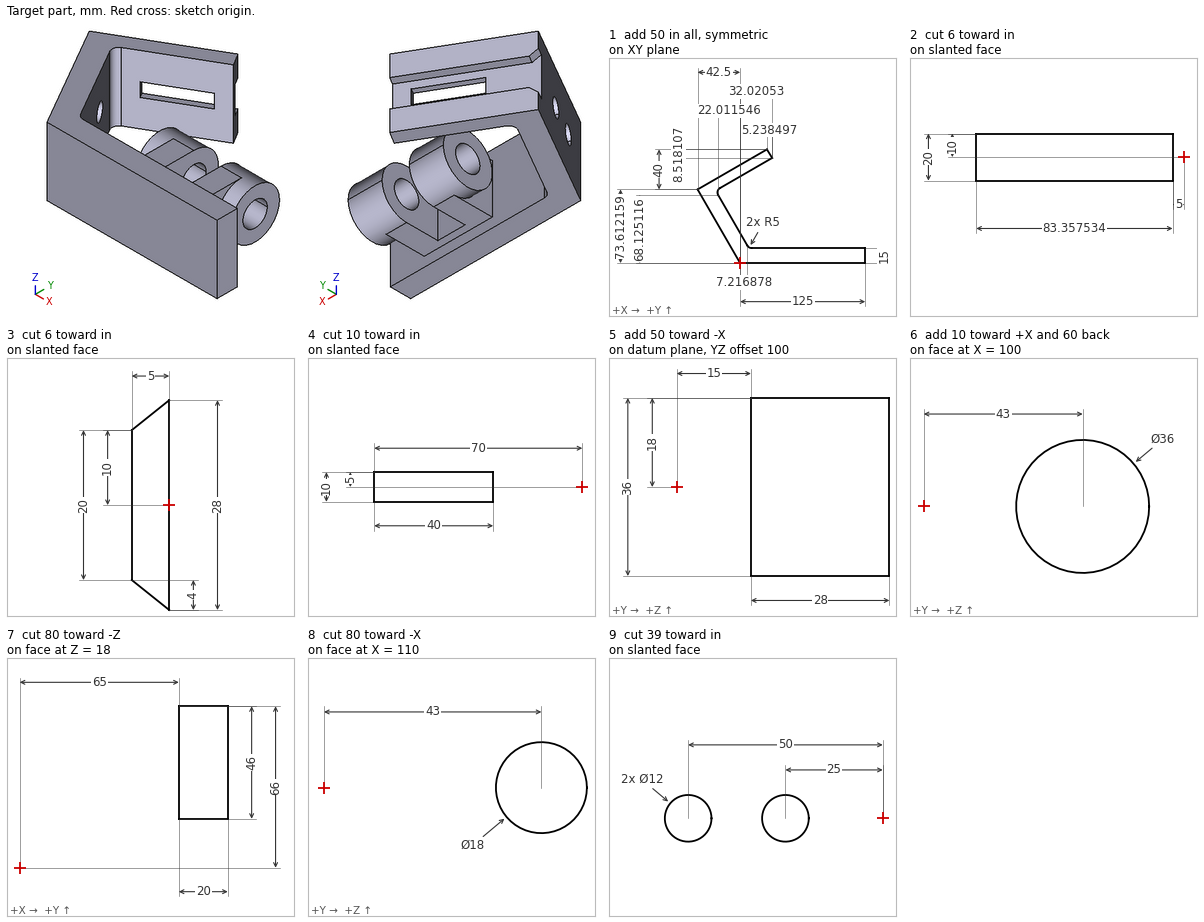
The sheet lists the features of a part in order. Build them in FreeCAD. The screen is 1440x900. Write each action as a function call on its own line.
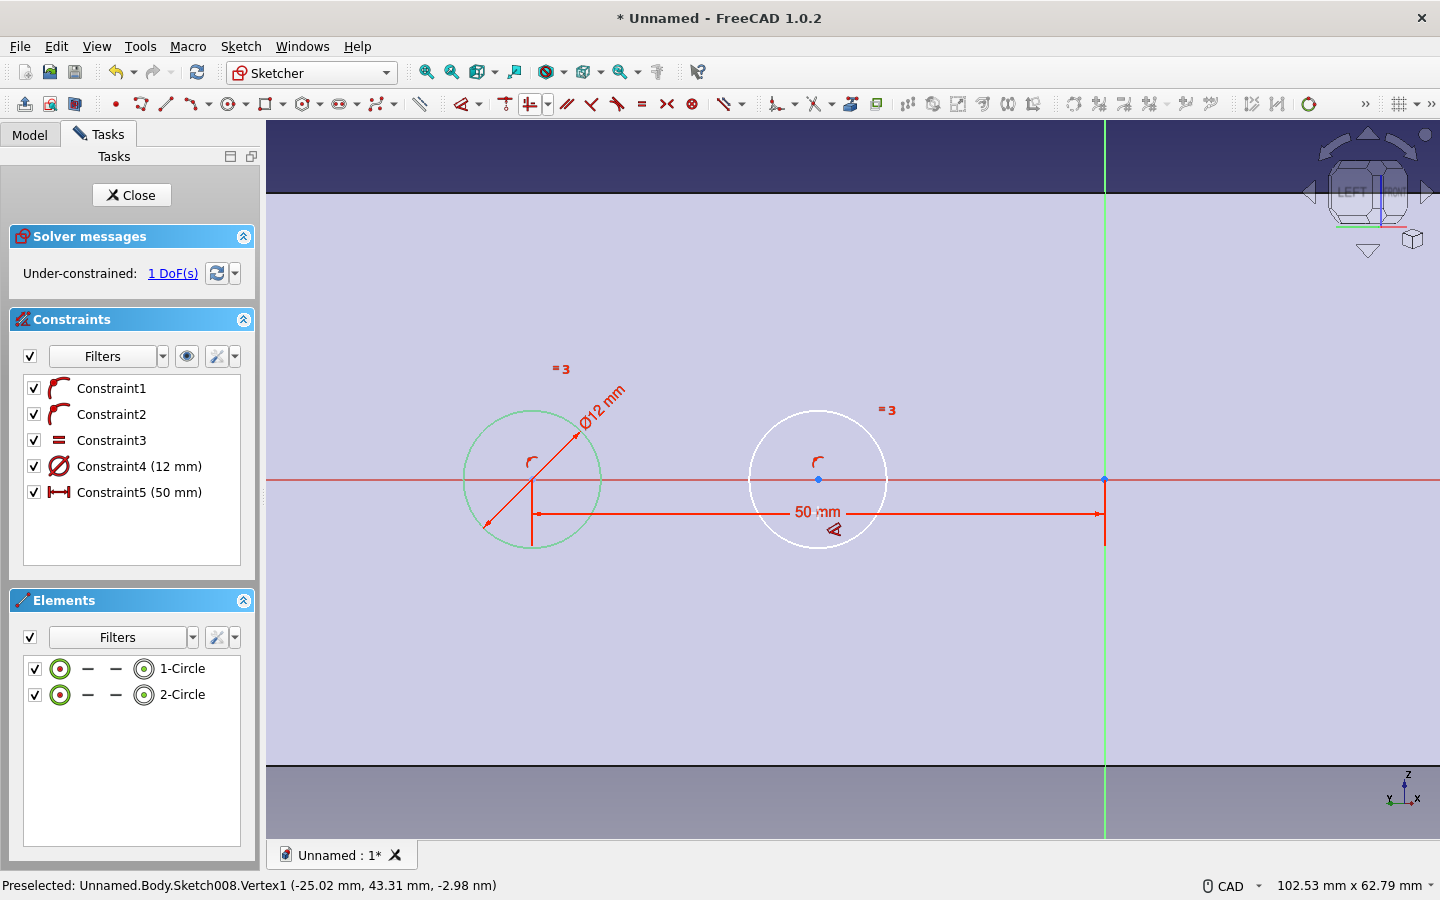
click(818, 479)
click(961, 513)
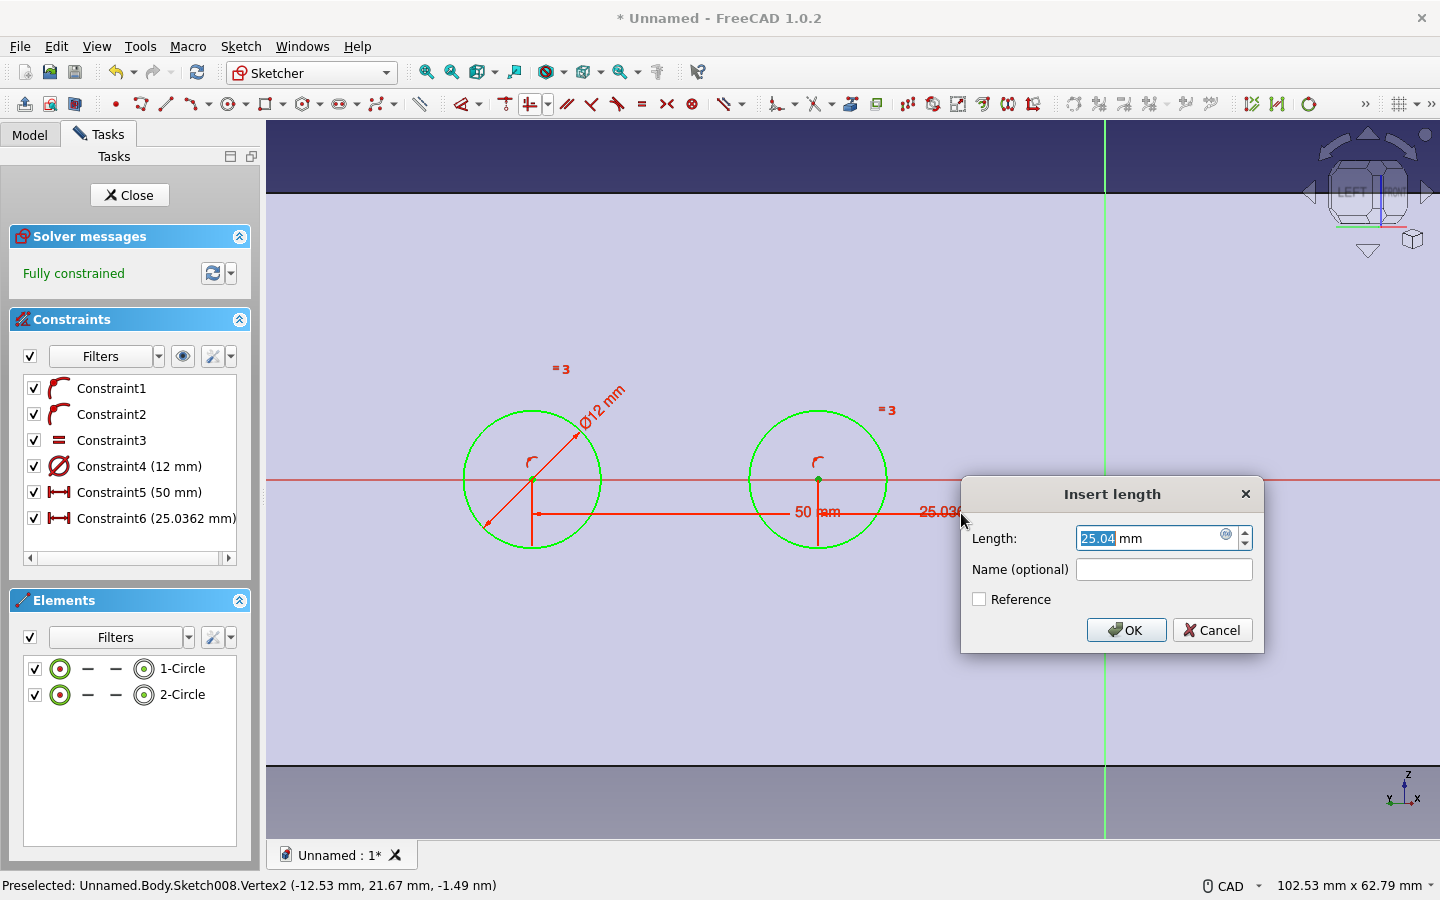
text(25)
key(Return)
key(Escape)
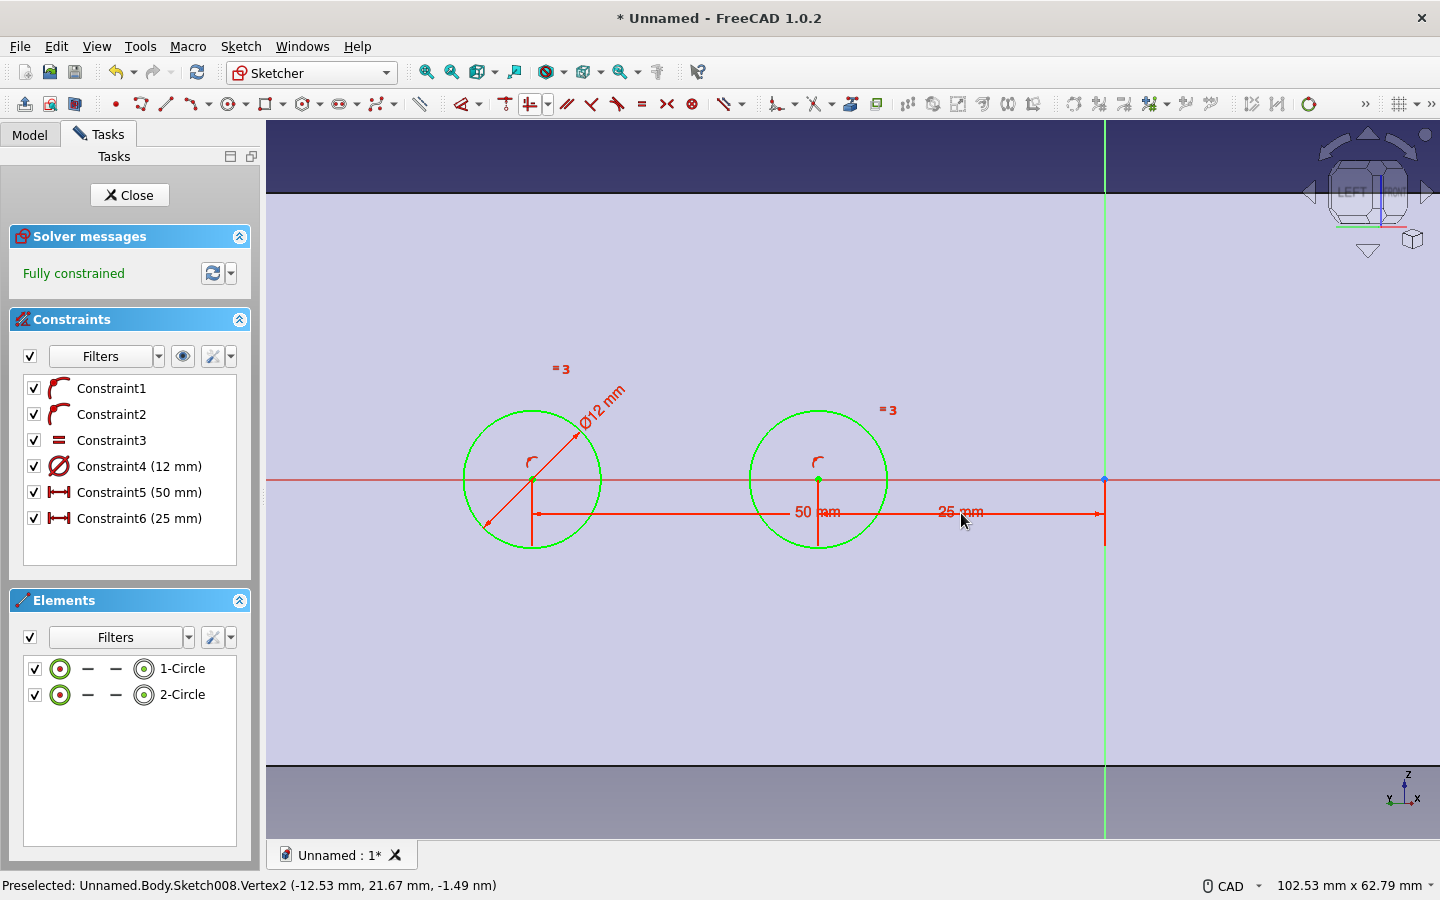
click(130, 195)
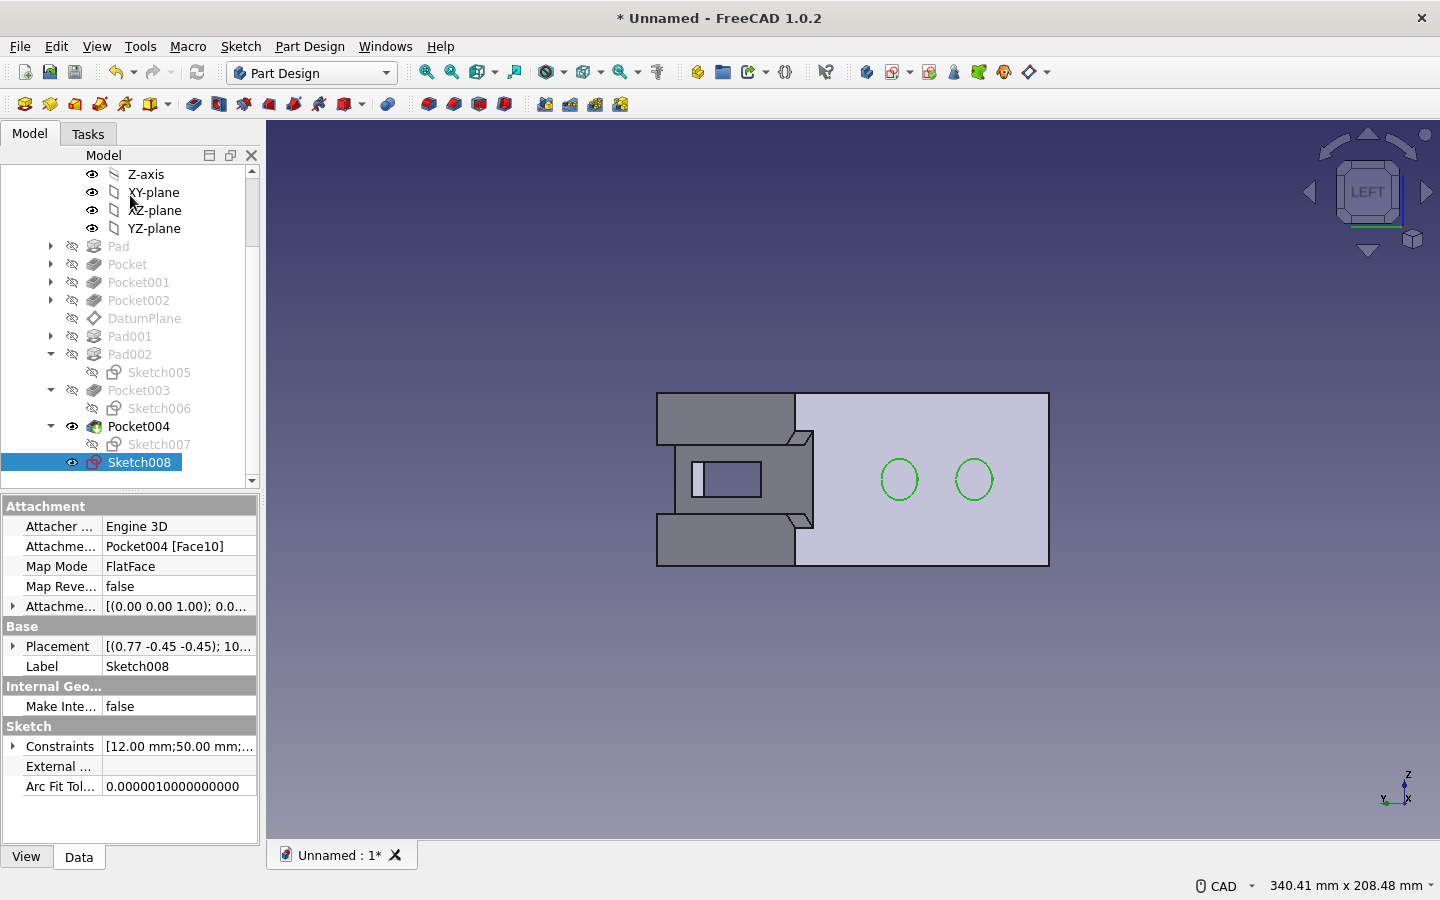
click(194, 104)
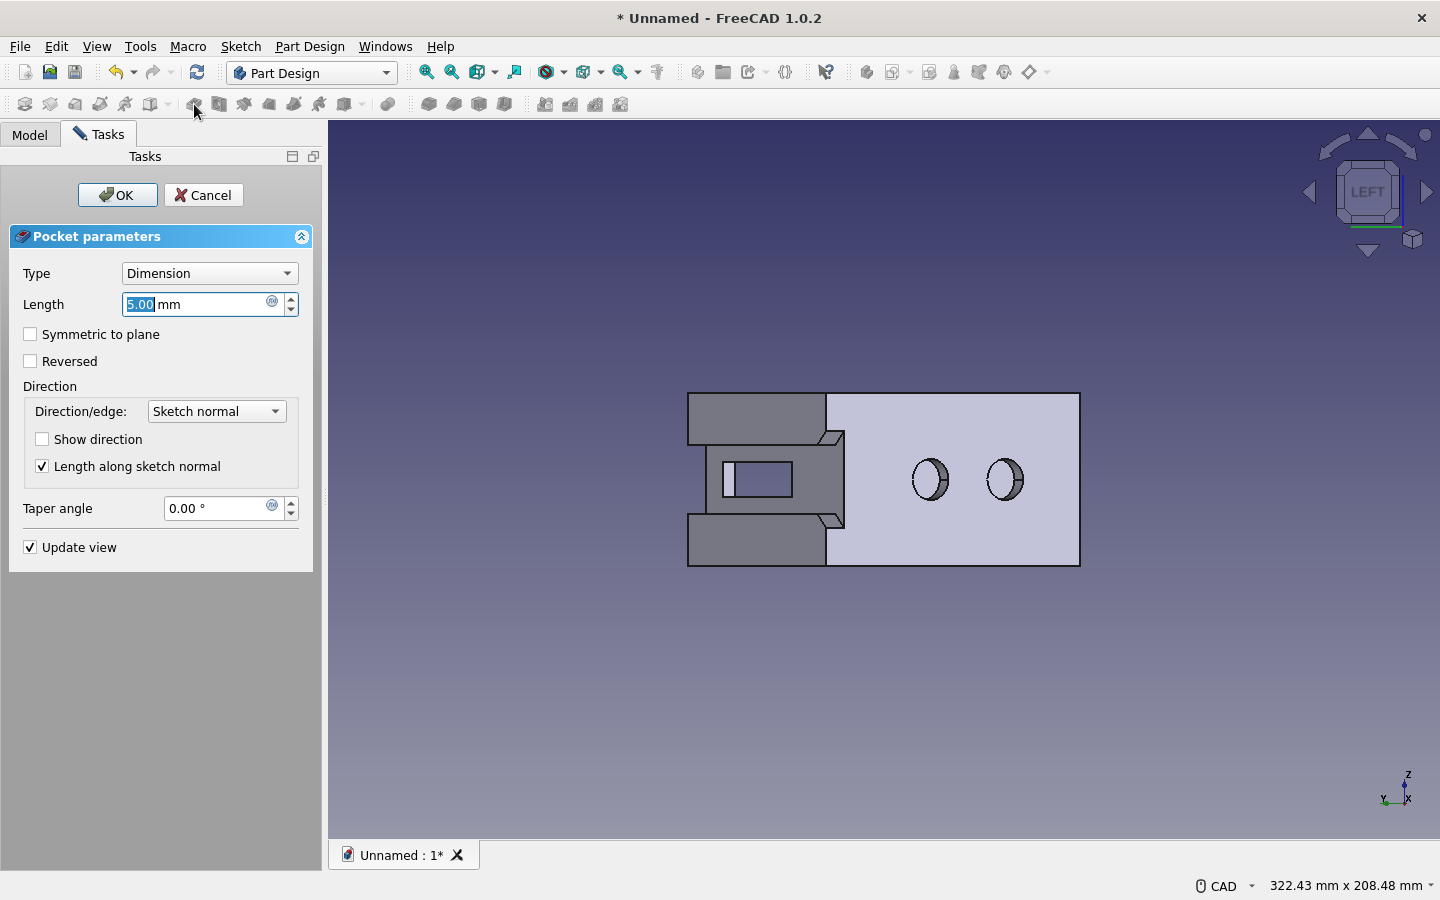
text(39)
key(Tab)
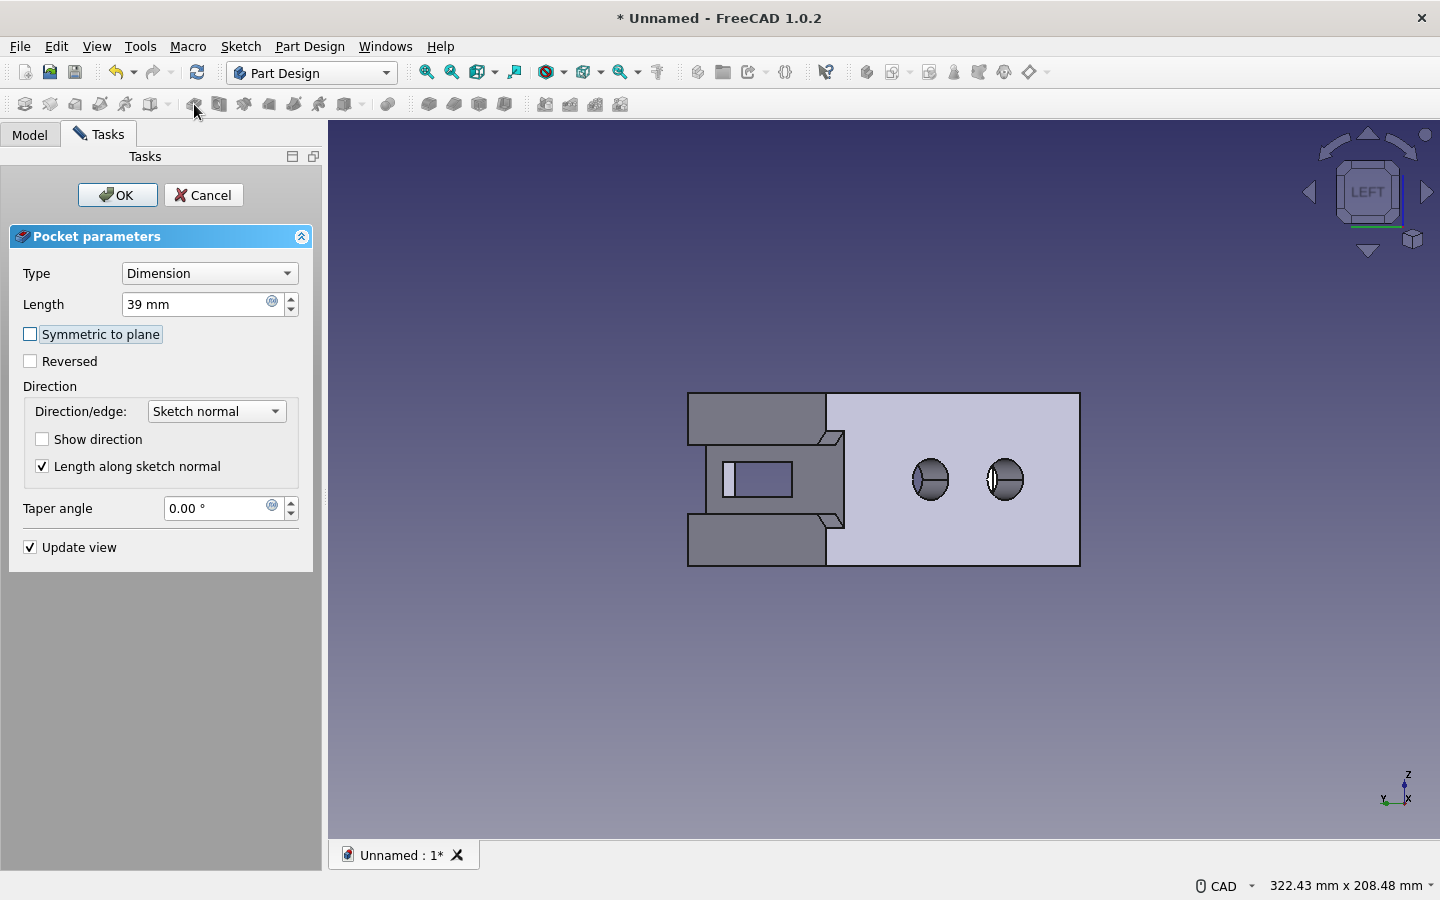
click(118, 195)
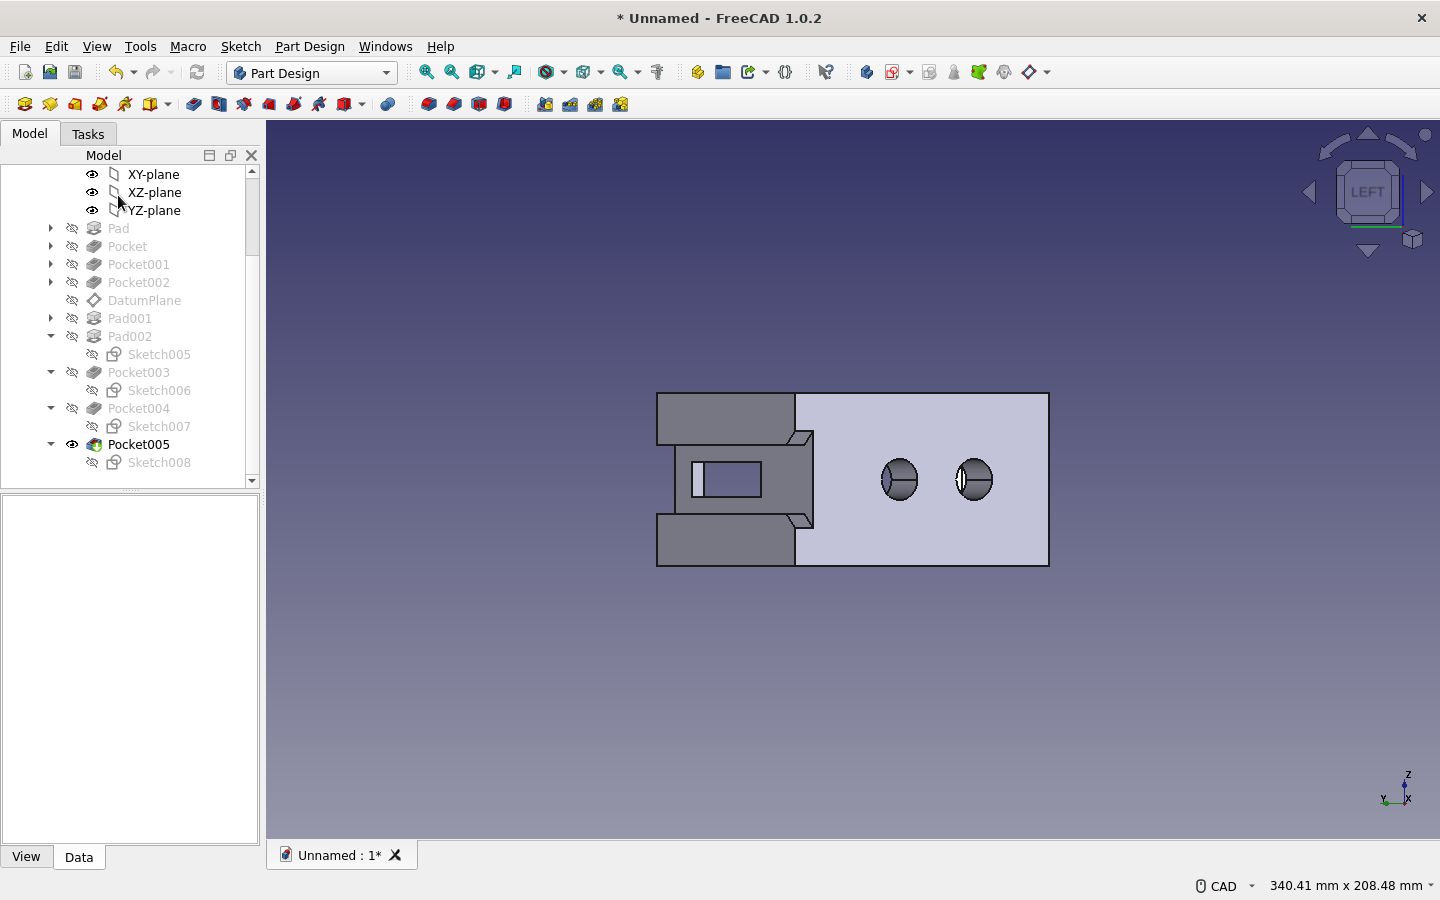
key(0)